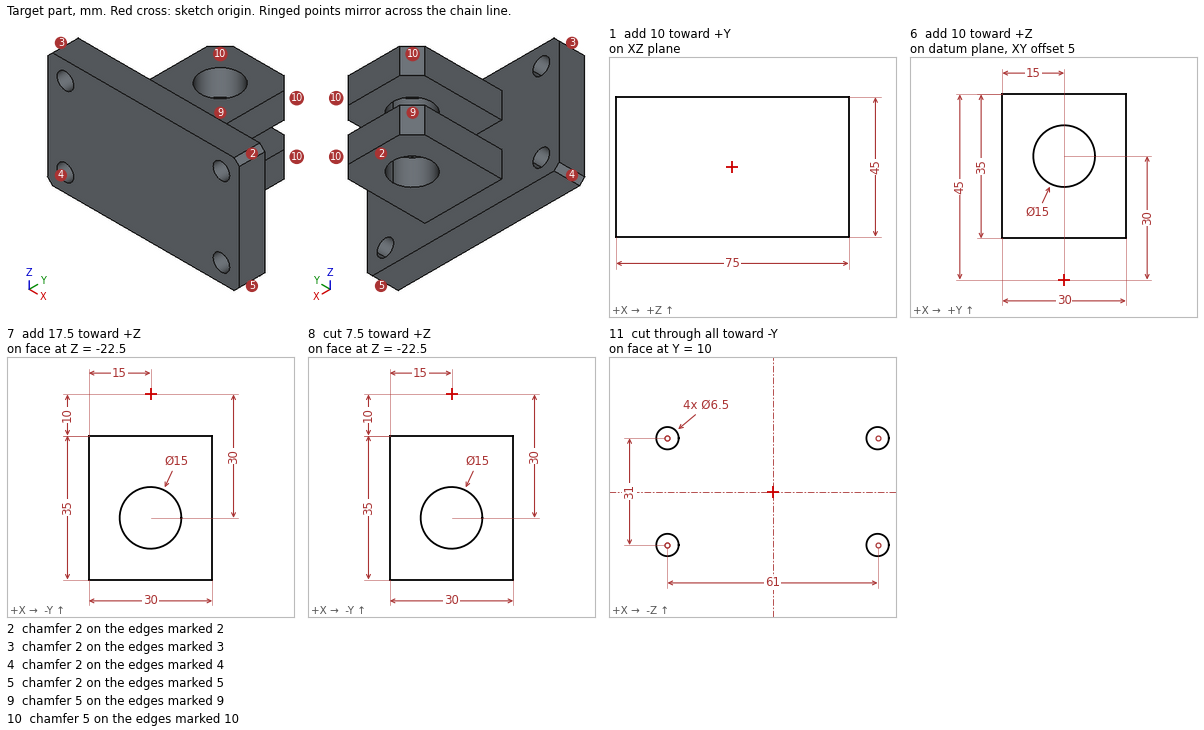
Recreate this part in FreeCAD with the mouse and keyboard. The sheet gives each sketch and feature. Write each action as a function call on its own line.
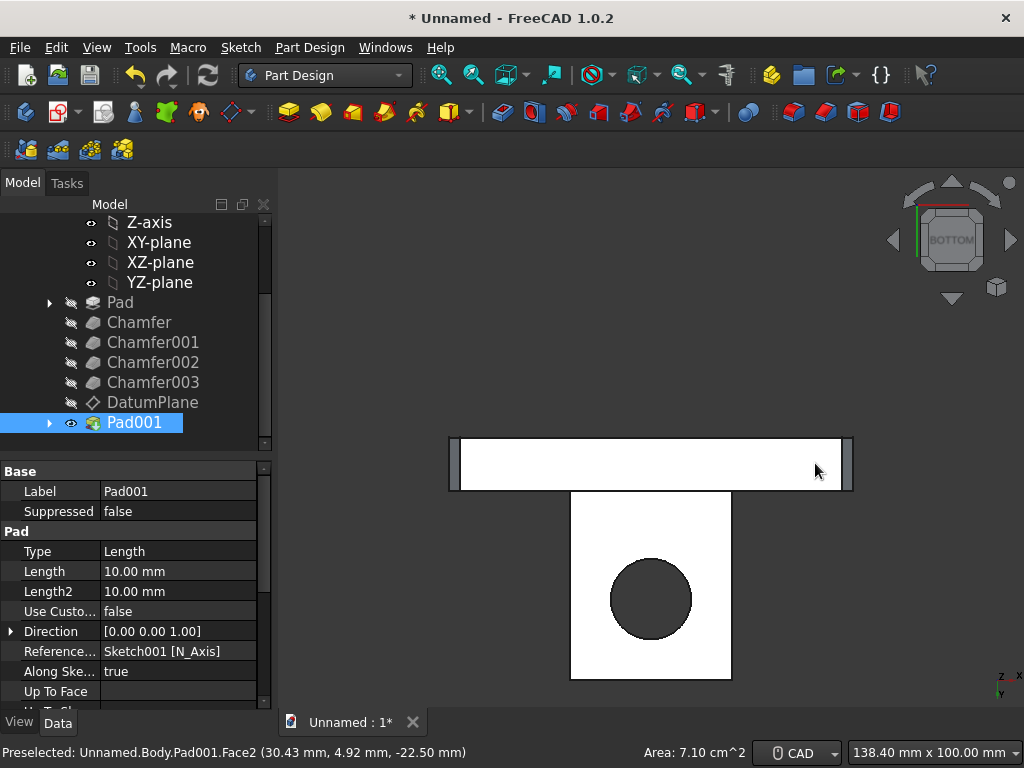
click(58, 112)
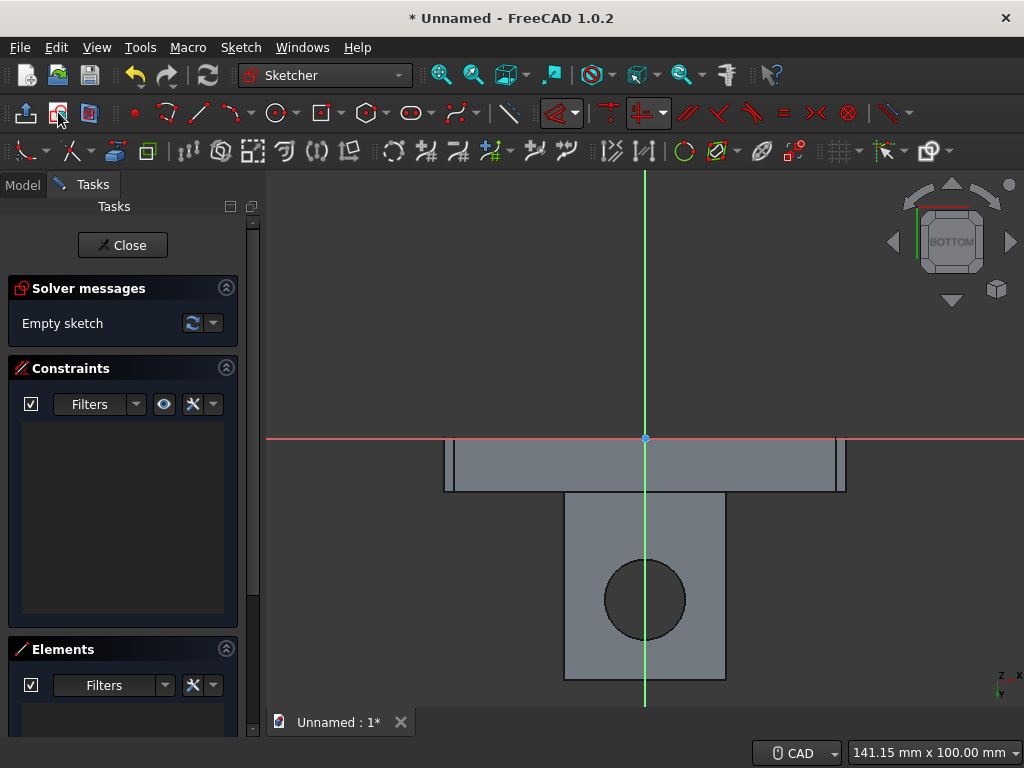
scroll(294, 198, down, 1)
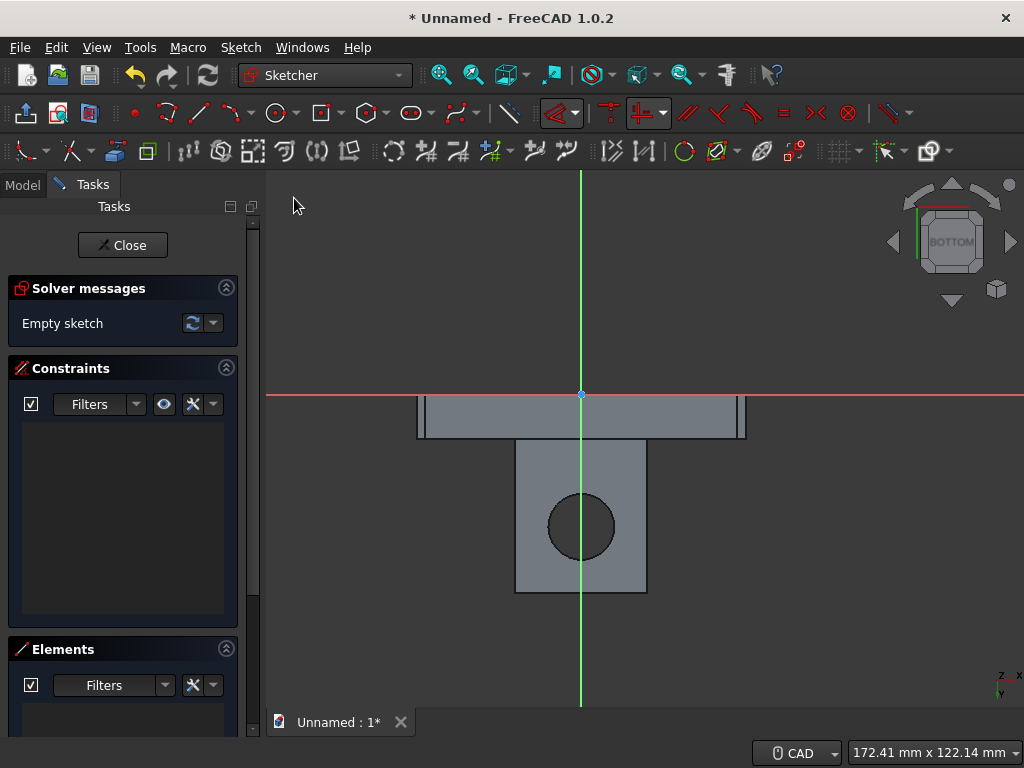
scroll(587, 561, up, 3)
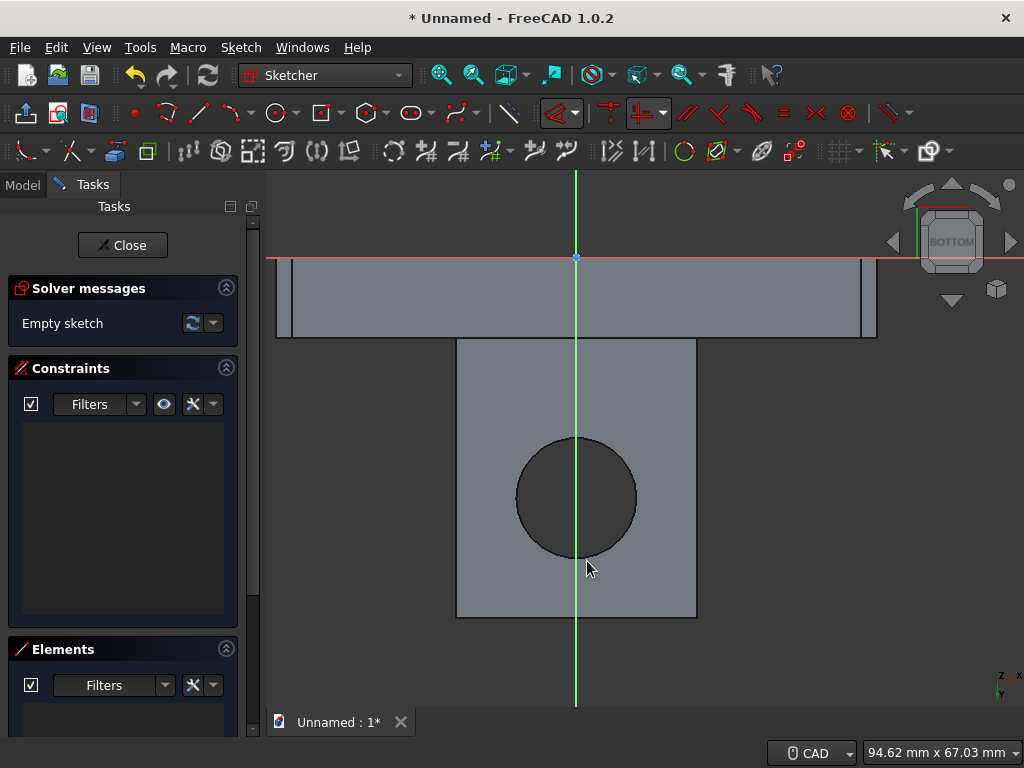
key(g)
key(r)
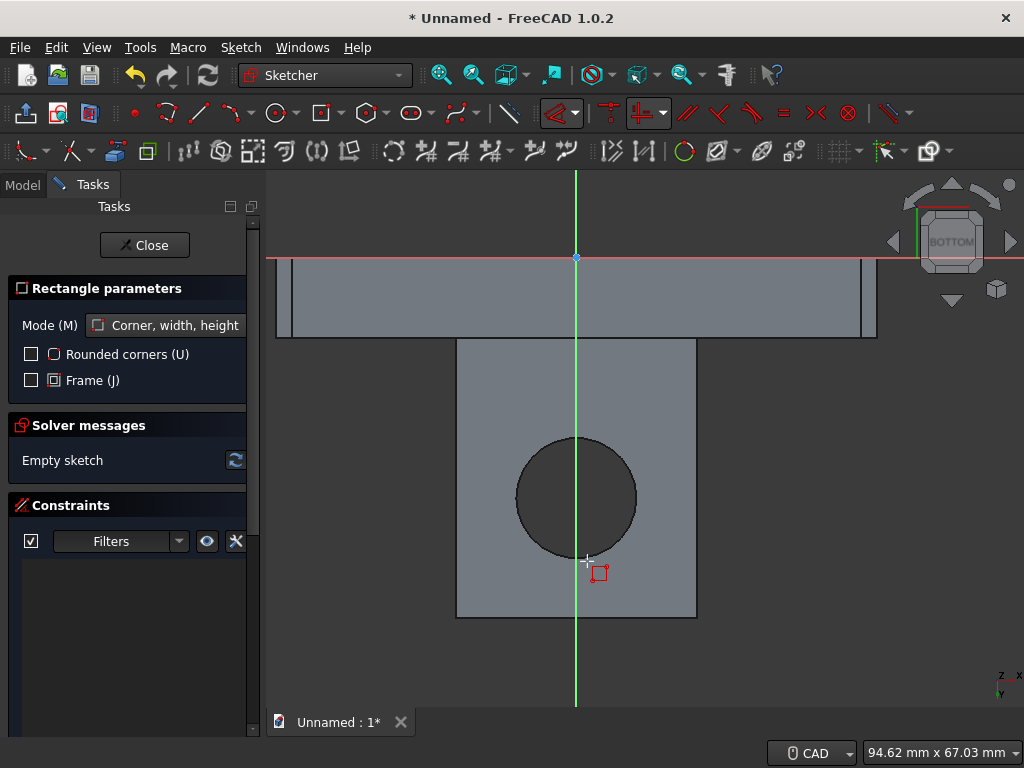
click(456, 338)
click(697, 618)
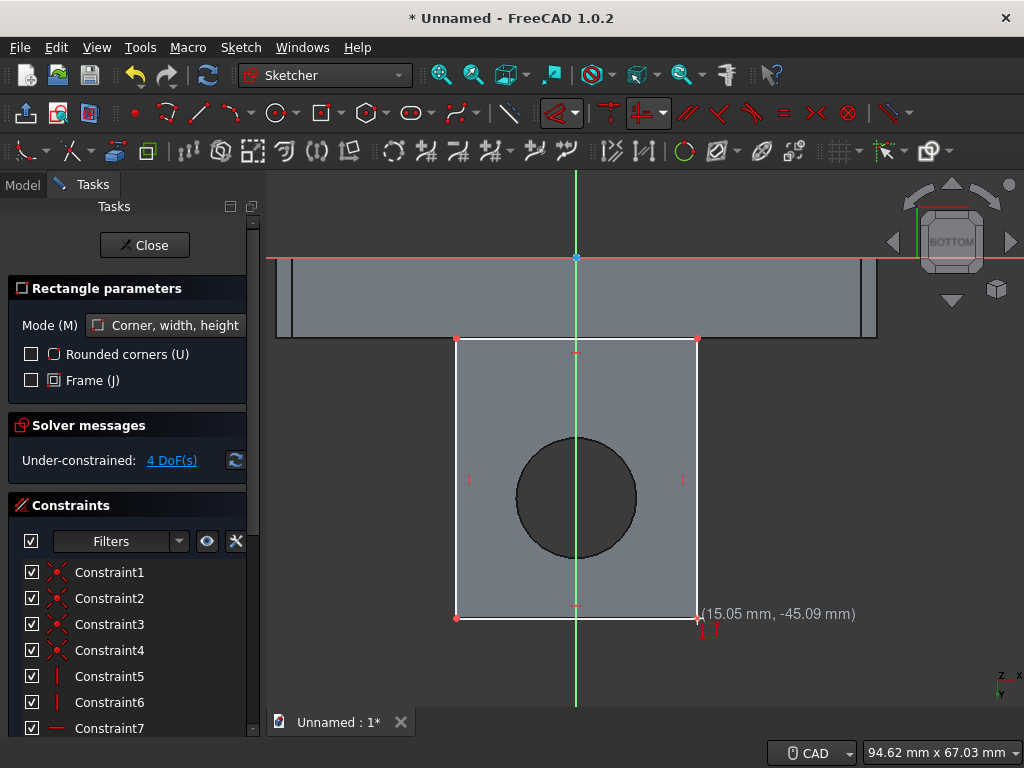
key(g)
key(c)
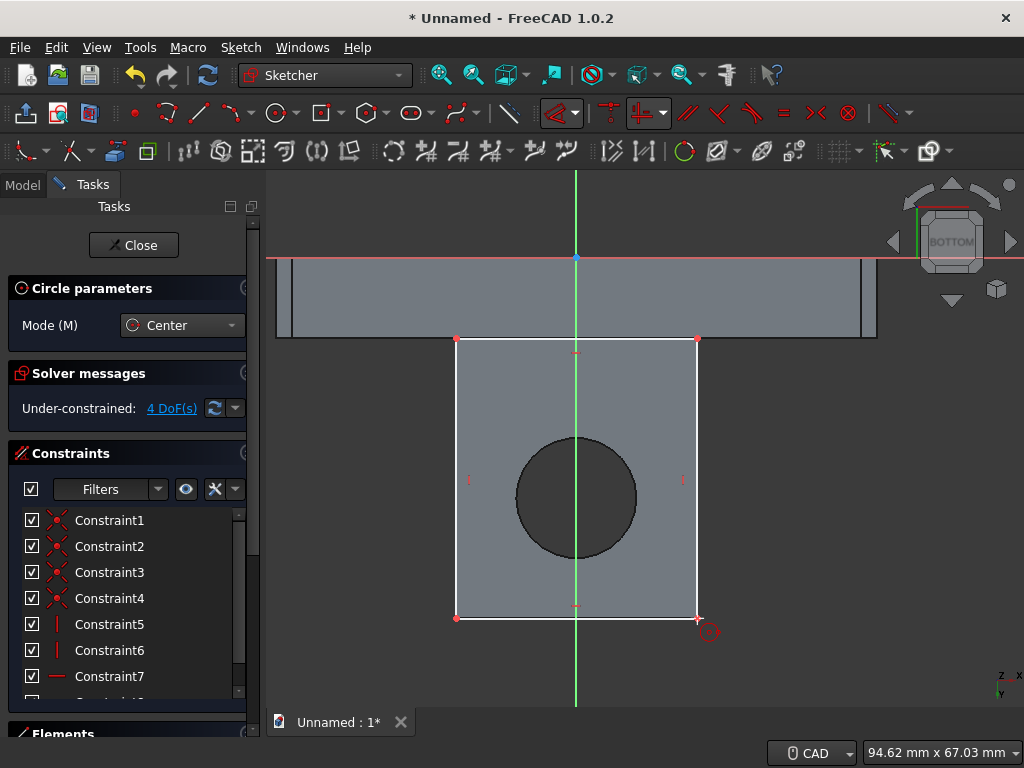
click(576, 498)
click(619, 456)
key(Escape)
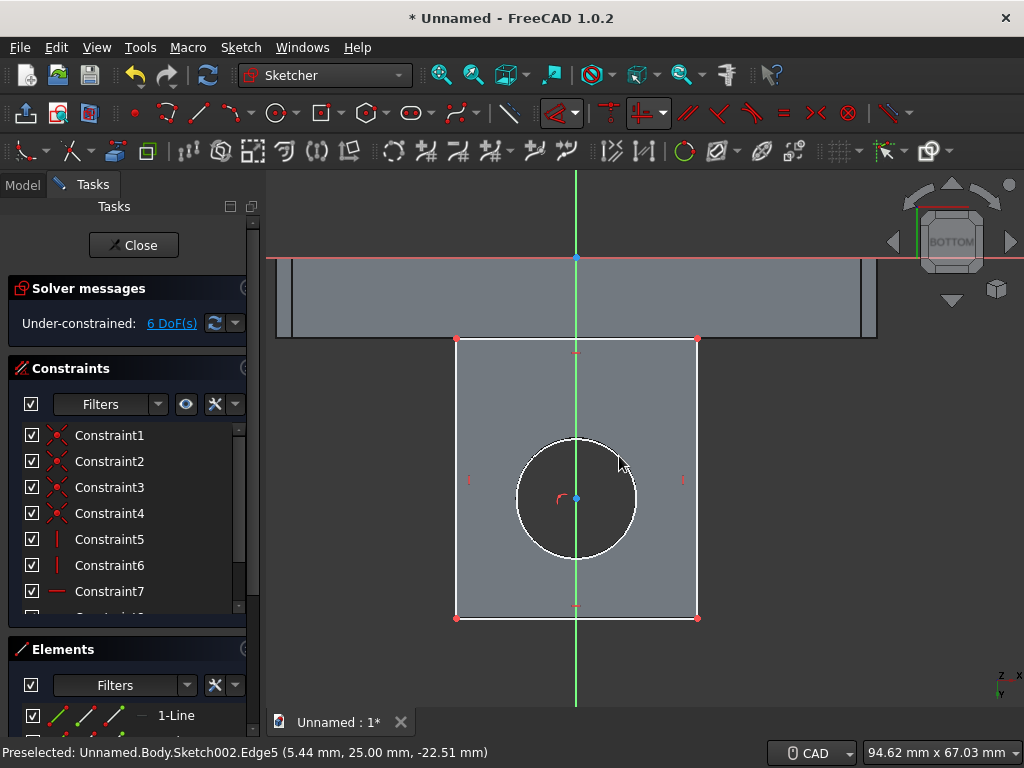
key(d)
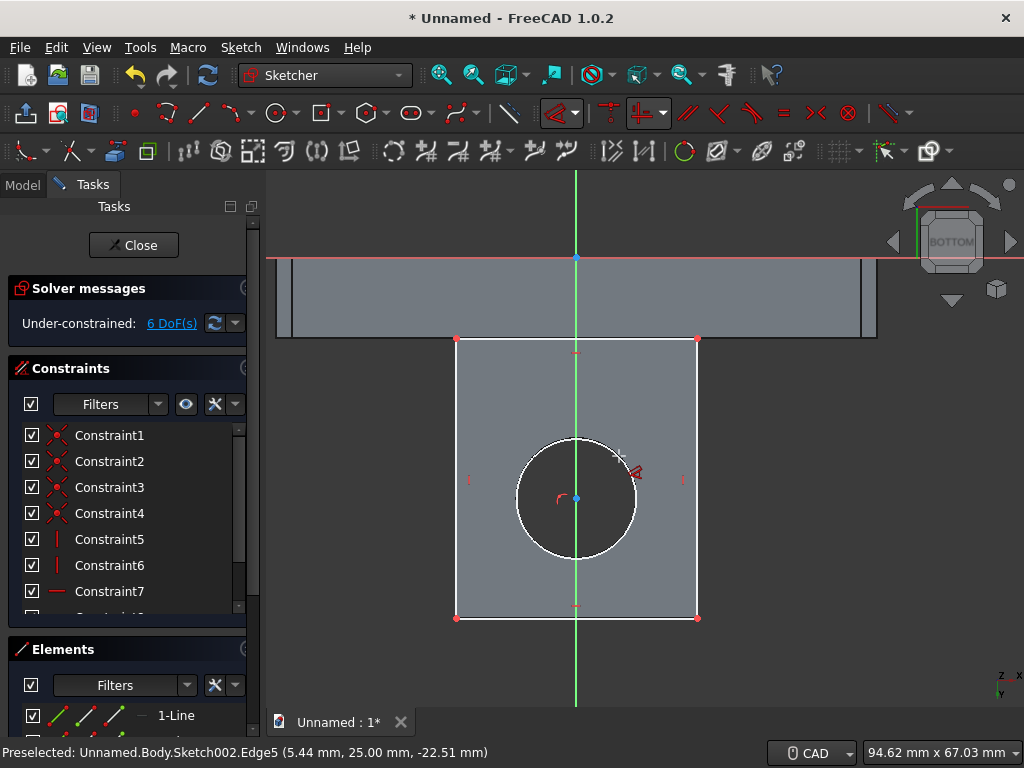
click(619, 457)
click(642, 435)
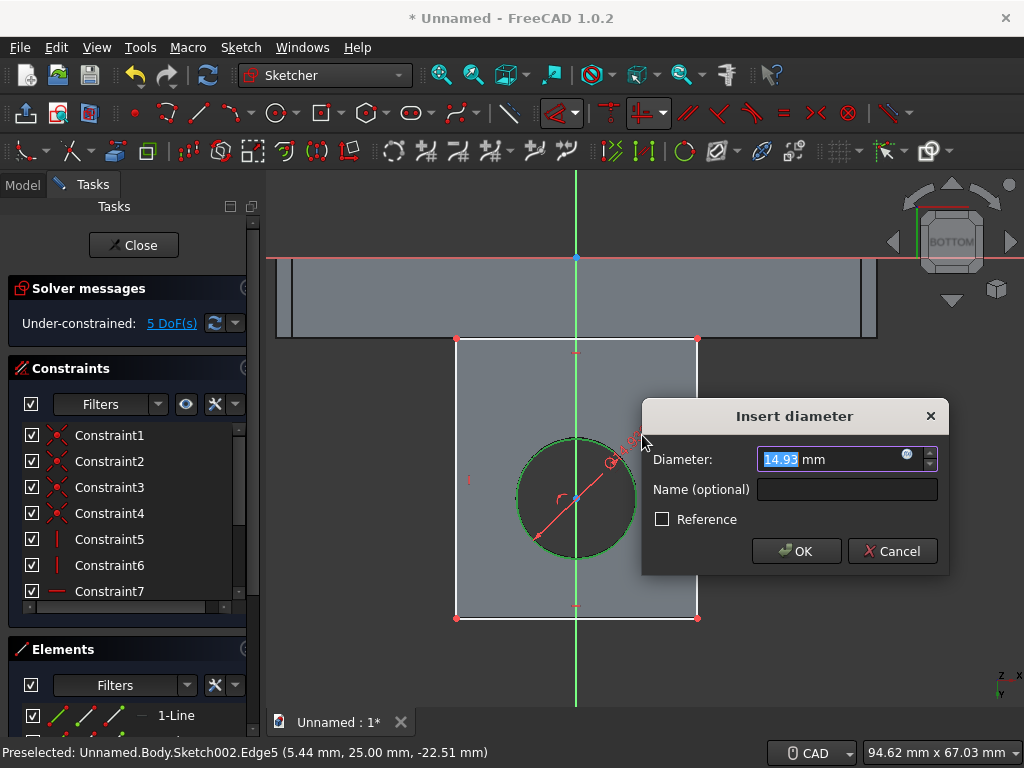
text(15)
key(Return)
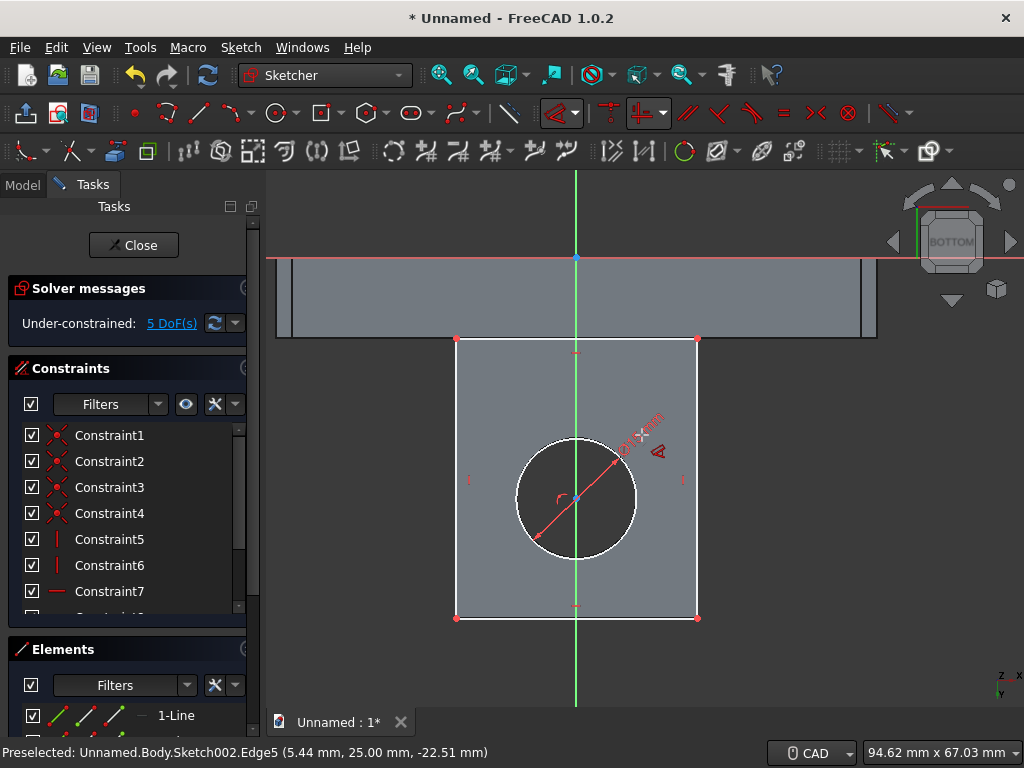
click(456, 423)
click(422, 479)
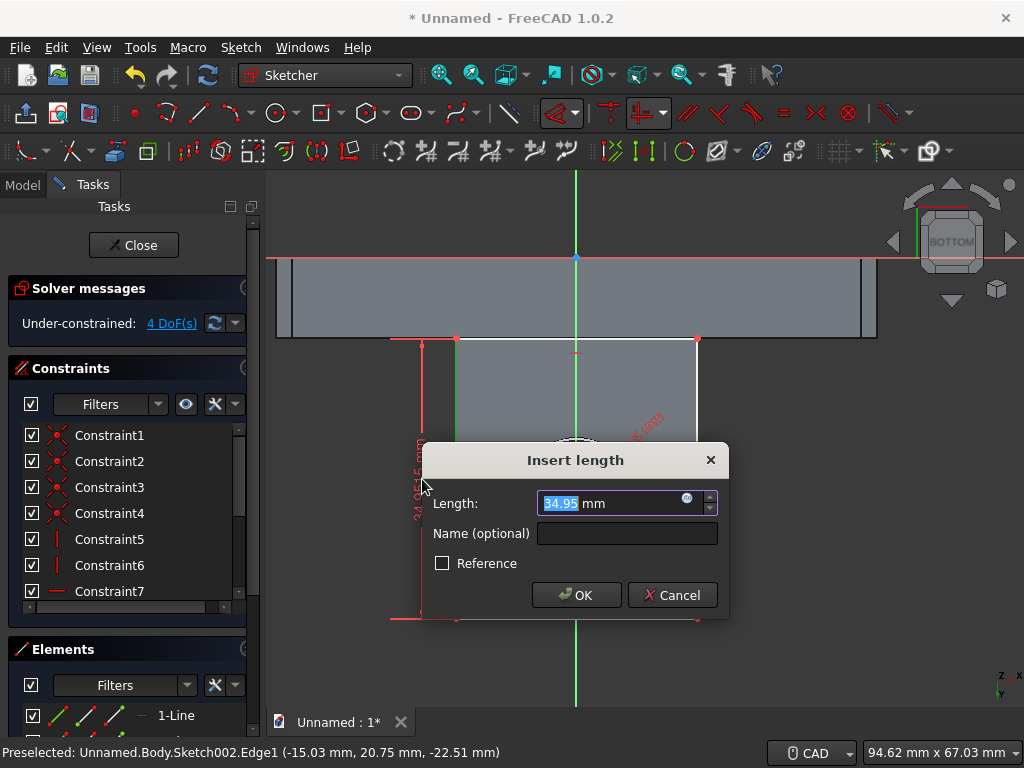
text(35)
key(Return)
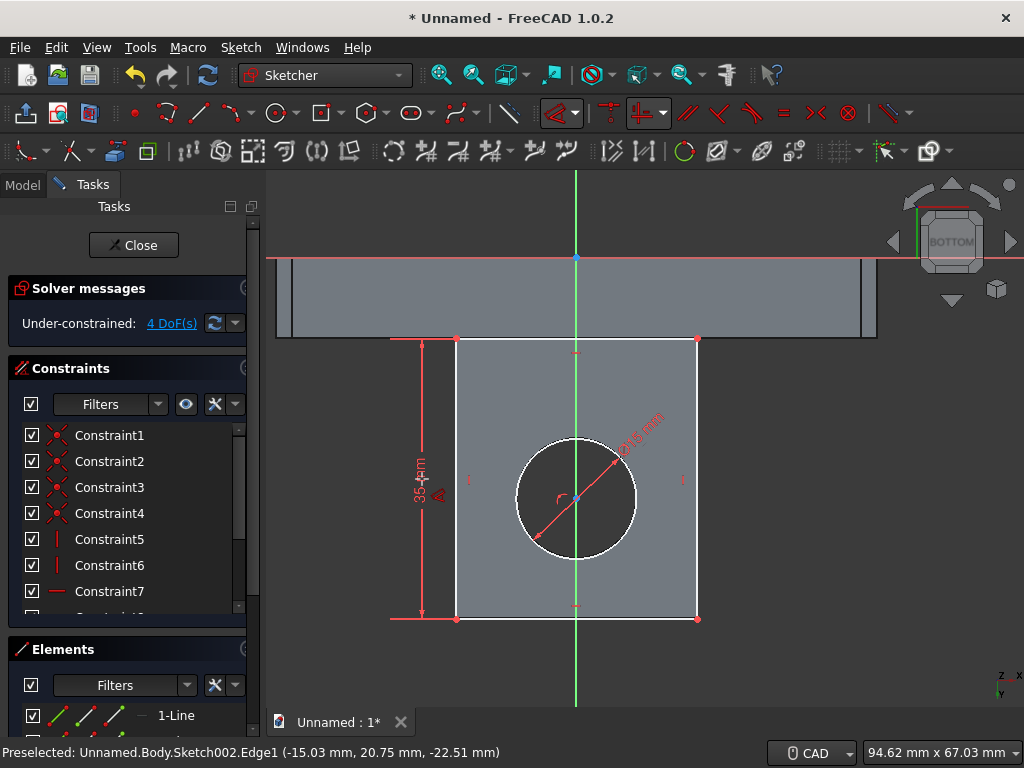
click(528, 619)
click(521, 653)